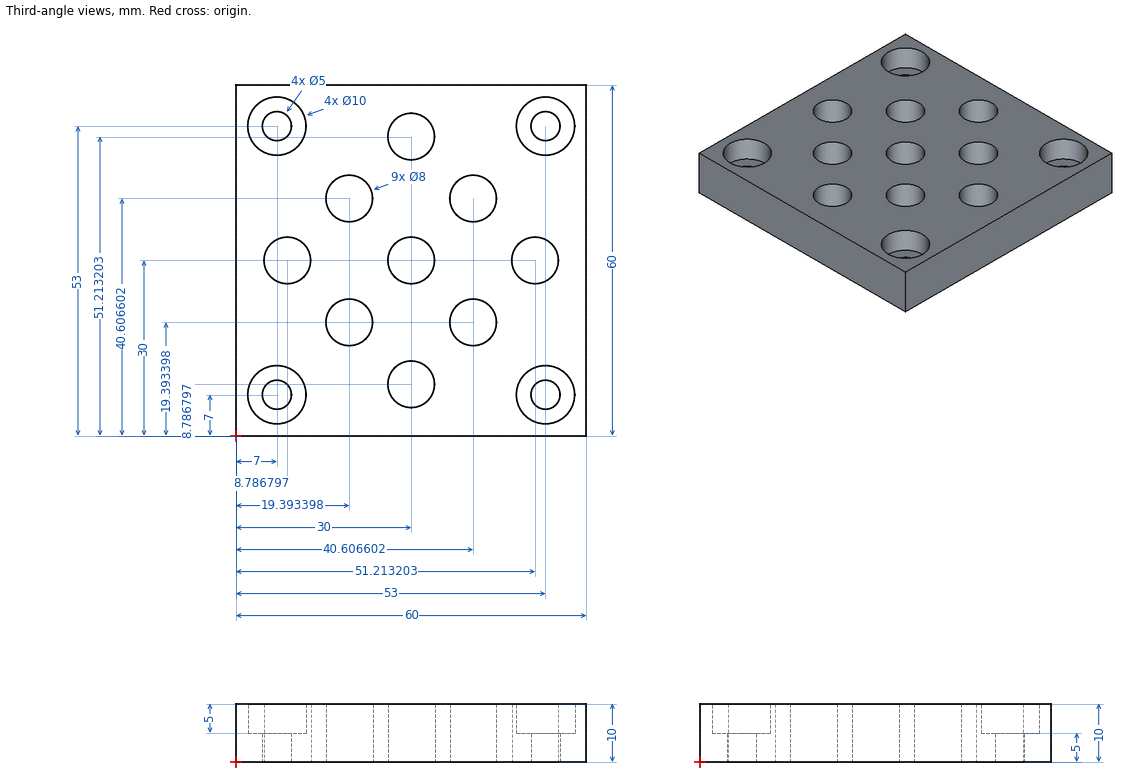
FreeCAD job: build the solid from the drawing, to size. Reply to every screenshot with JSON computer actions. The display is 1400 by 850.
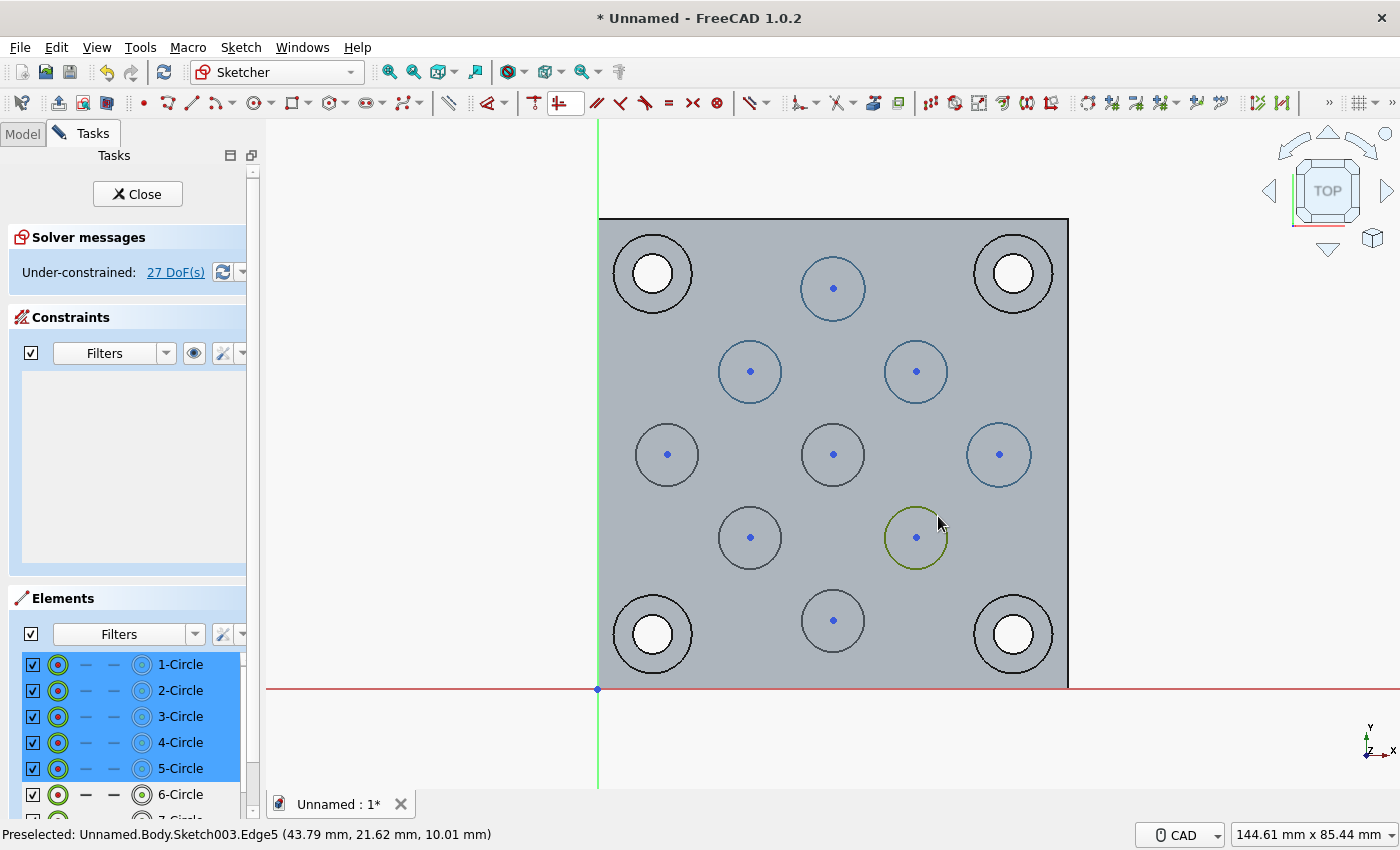
{"action": "left_click", "coordinate": [772, 516]}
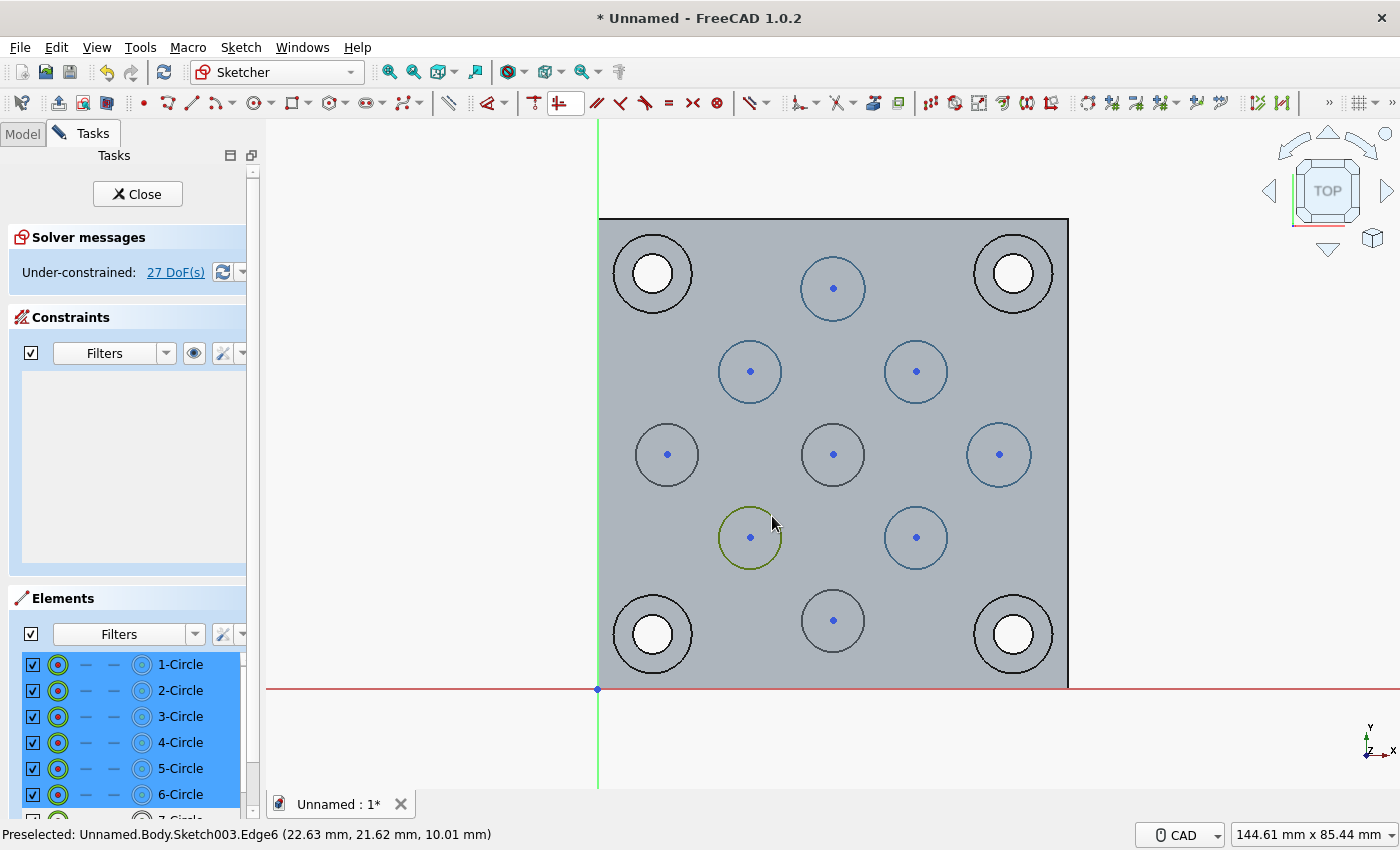
{"action": "left_click", "coordinate": [689, 433]}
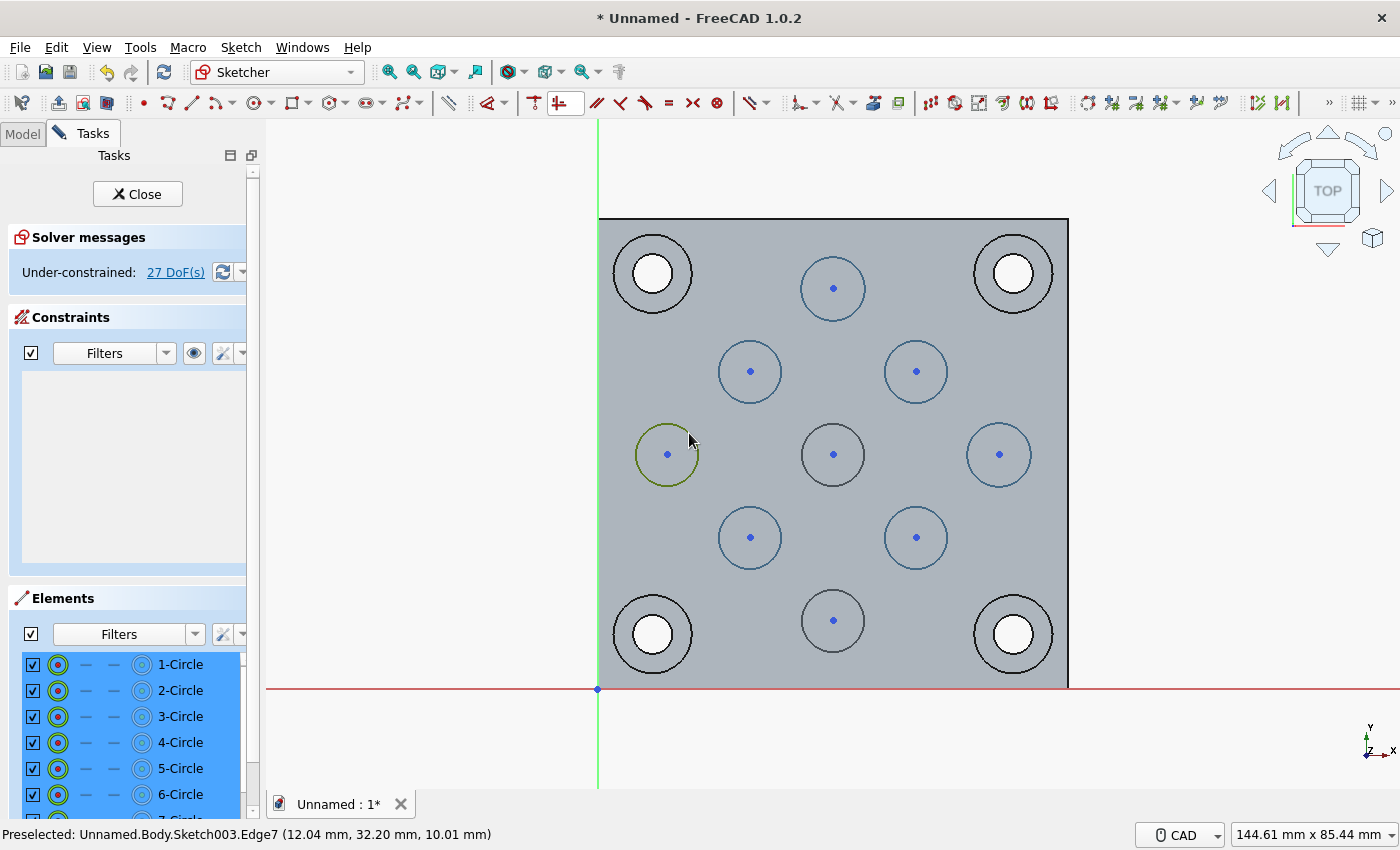
{"action": "left_click", "coordinate": [855, 599]}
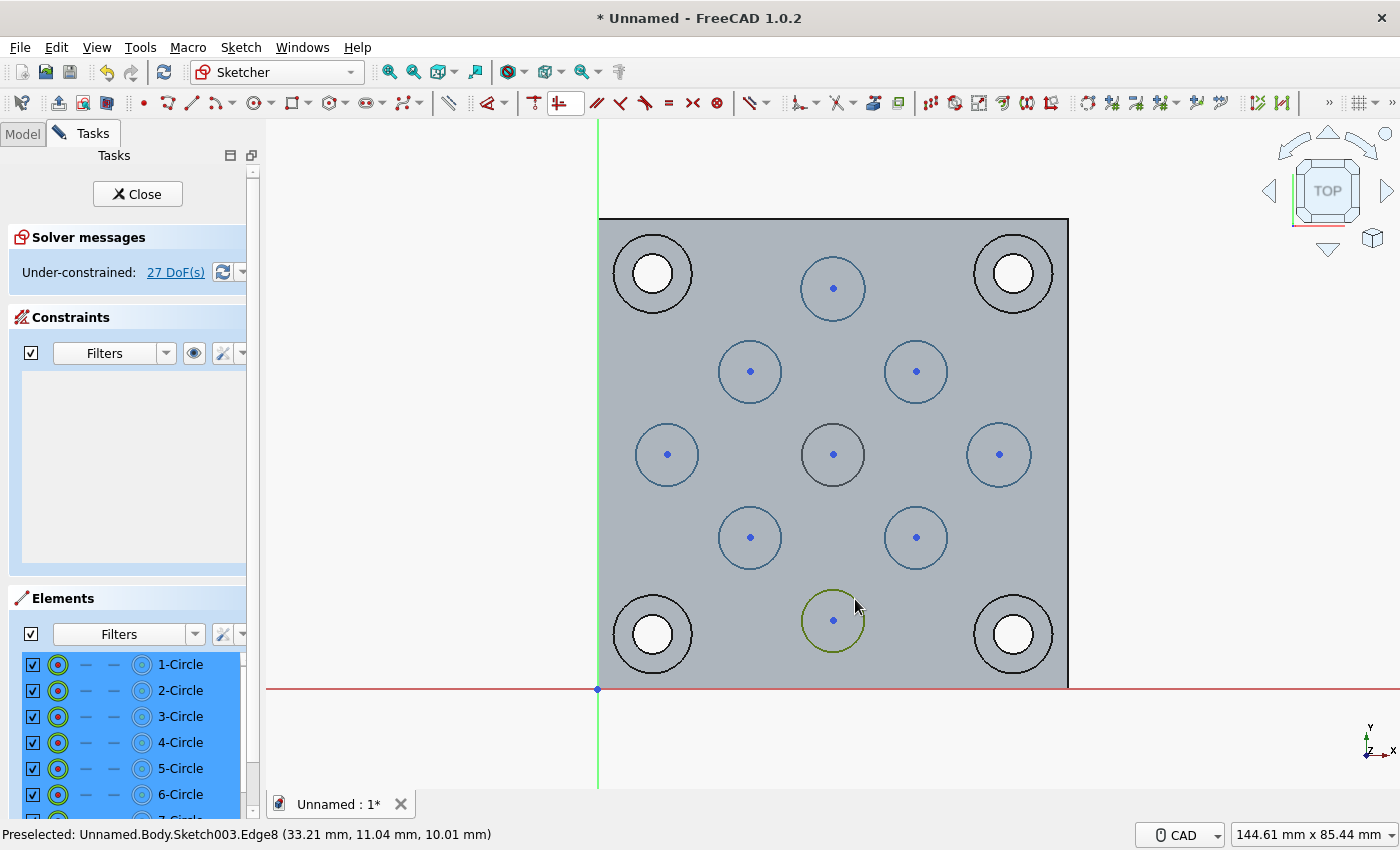
{"action": "left_click", "coordinate": [855, 433]}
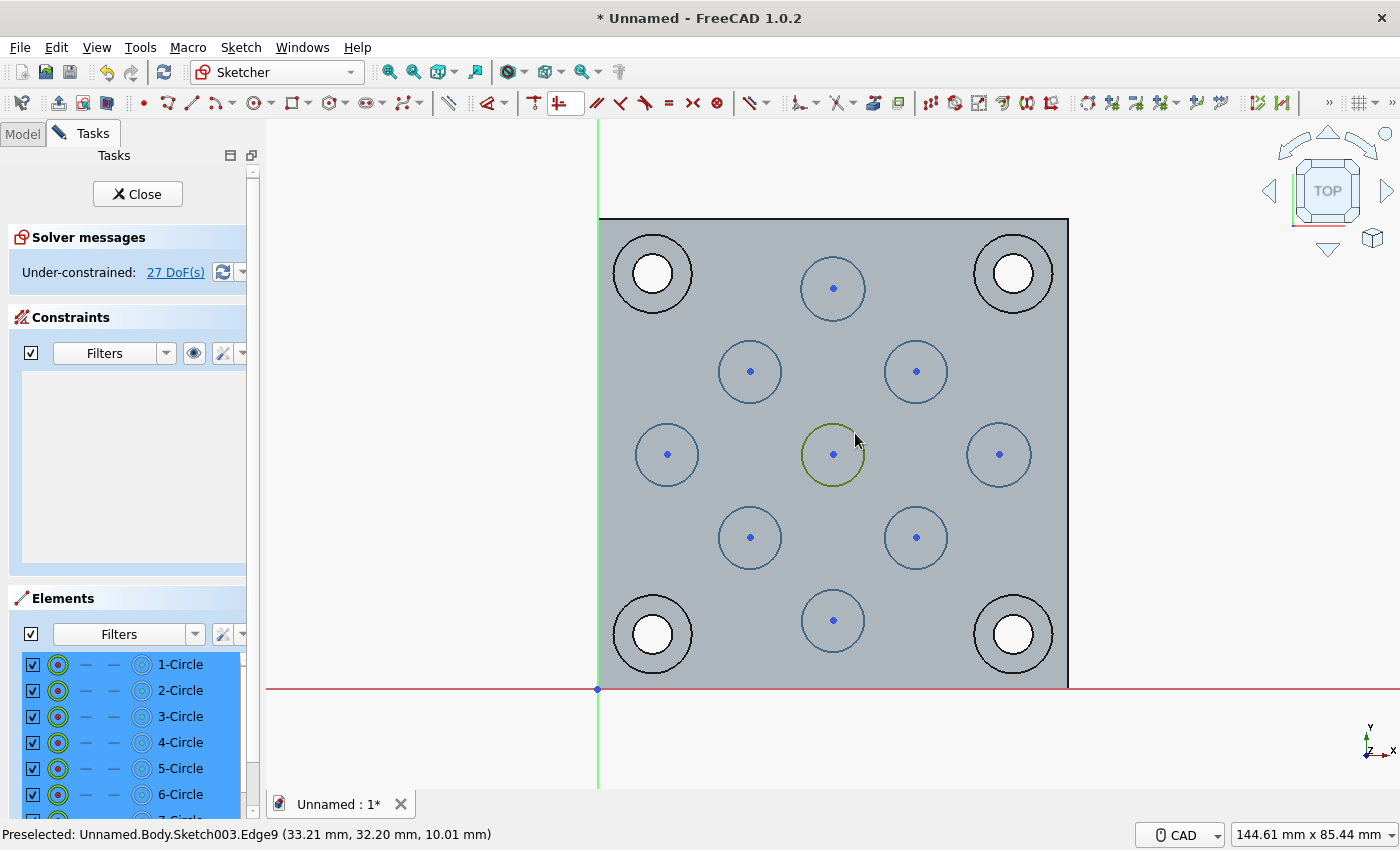
{"action": "left_click", "coordinate": [670, 104]}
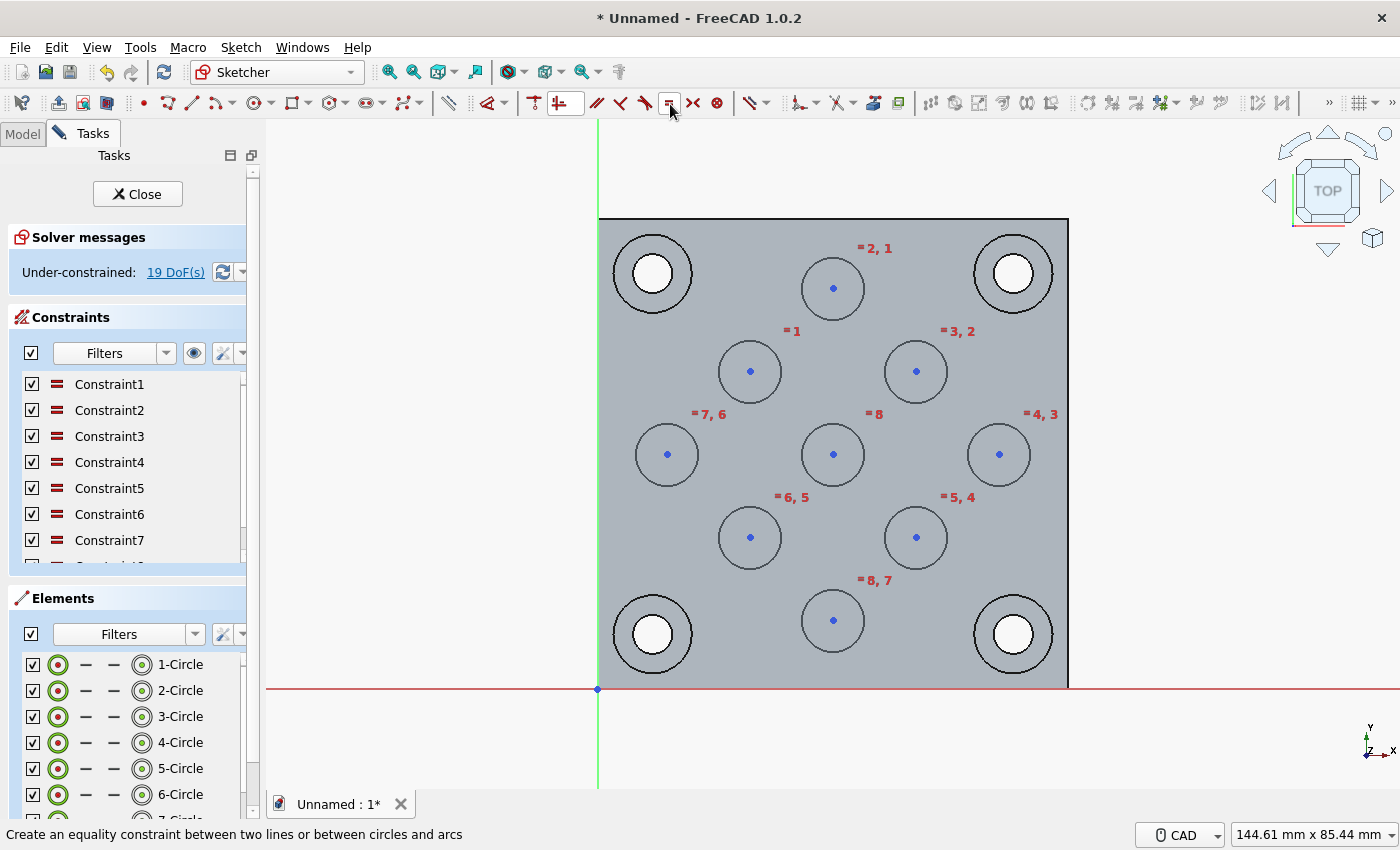
{"action": "left_click", "coordinate": [750, 372]}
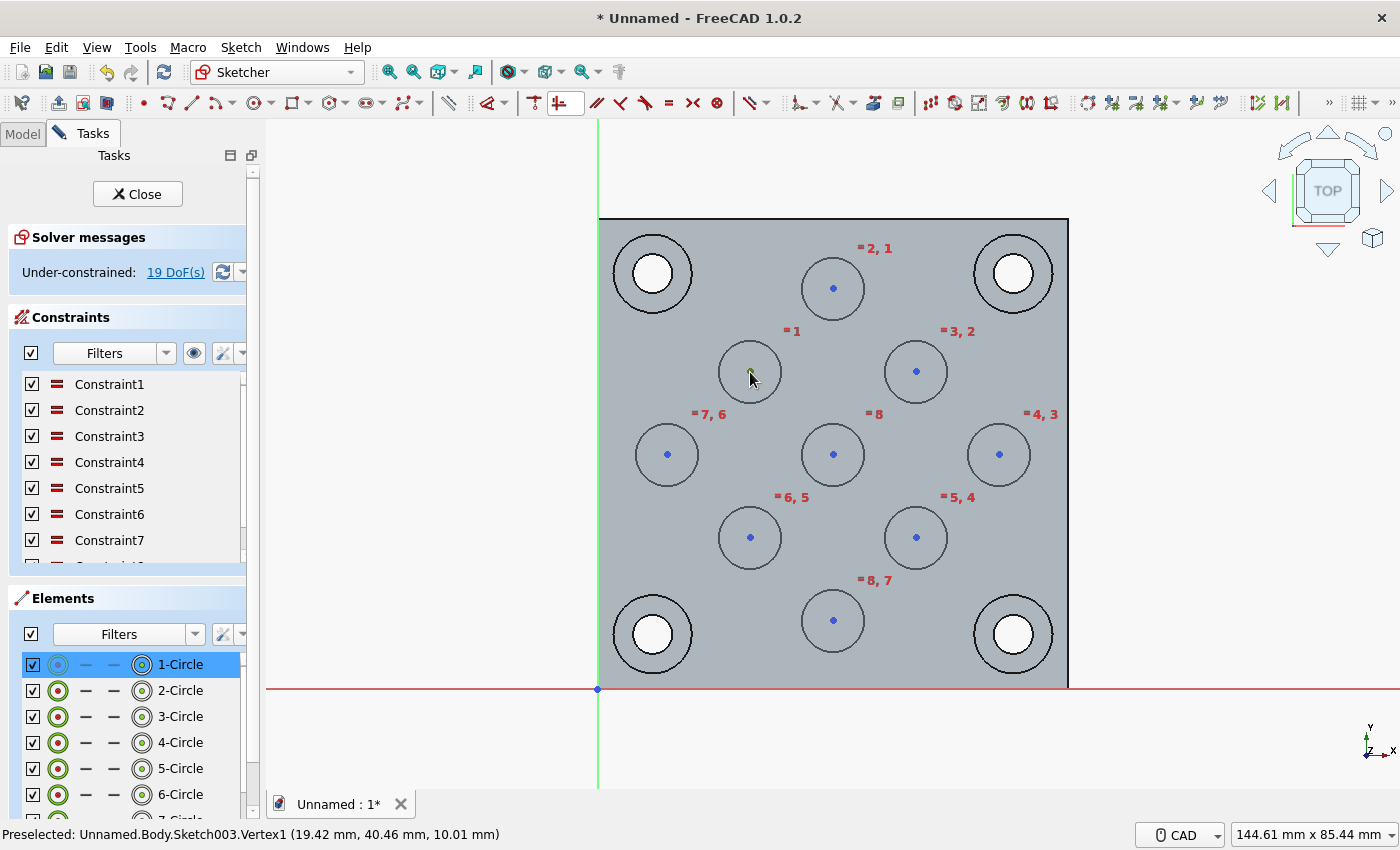
{"action": "left_click", "coordinate": [916, 372]}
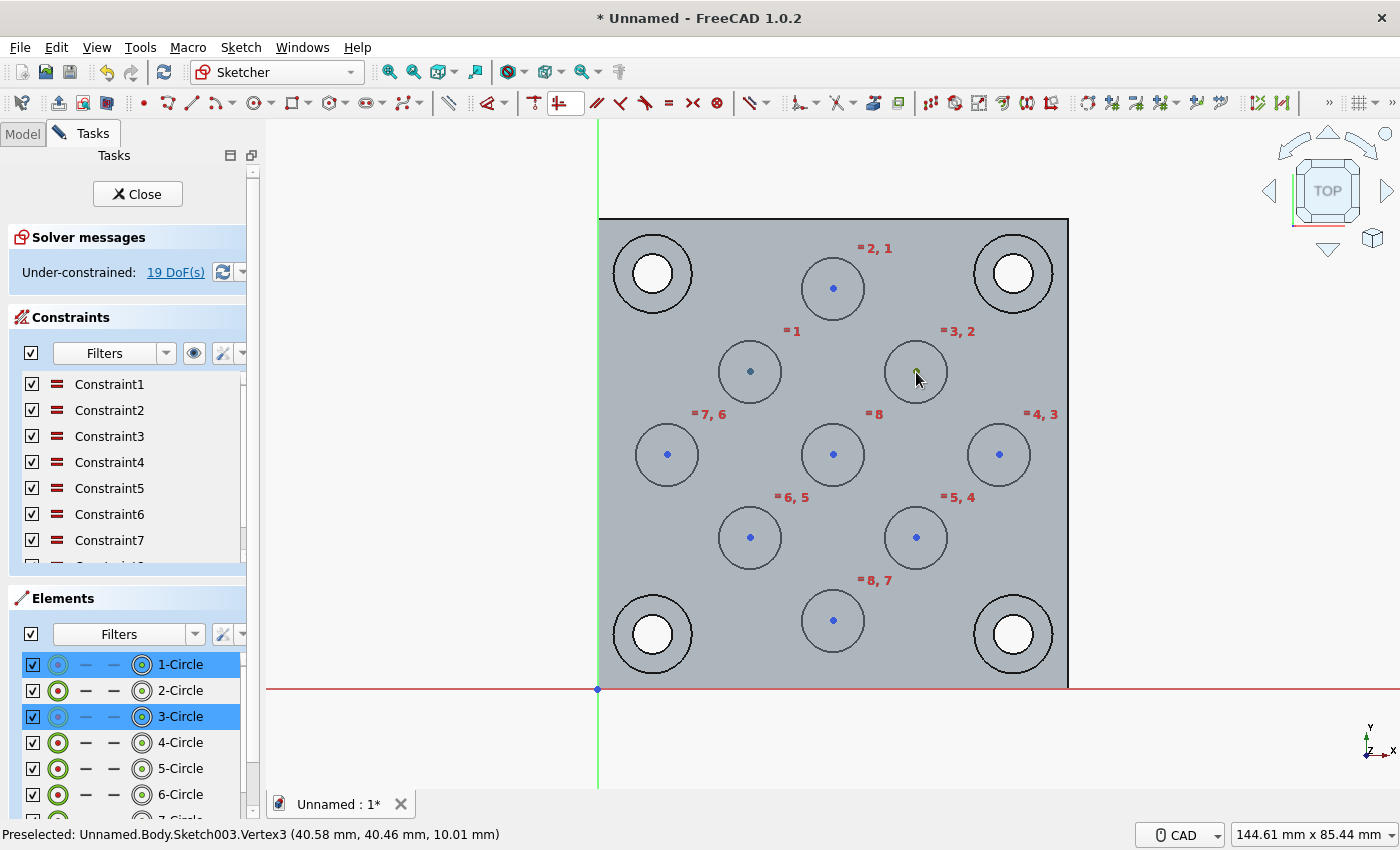
{"action": "left_click", "coordinate": [578, 104]}